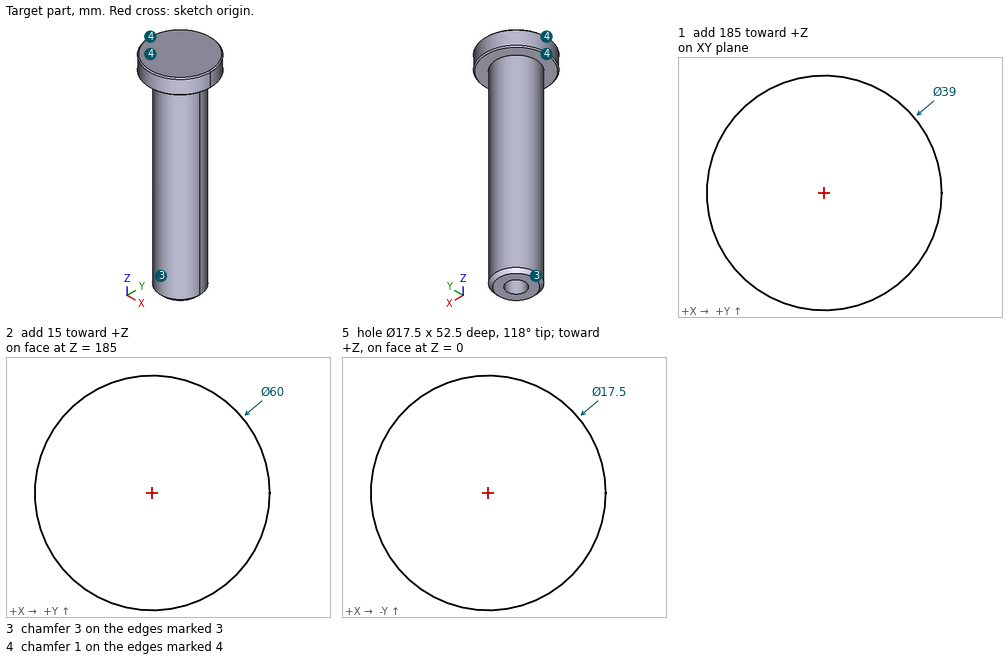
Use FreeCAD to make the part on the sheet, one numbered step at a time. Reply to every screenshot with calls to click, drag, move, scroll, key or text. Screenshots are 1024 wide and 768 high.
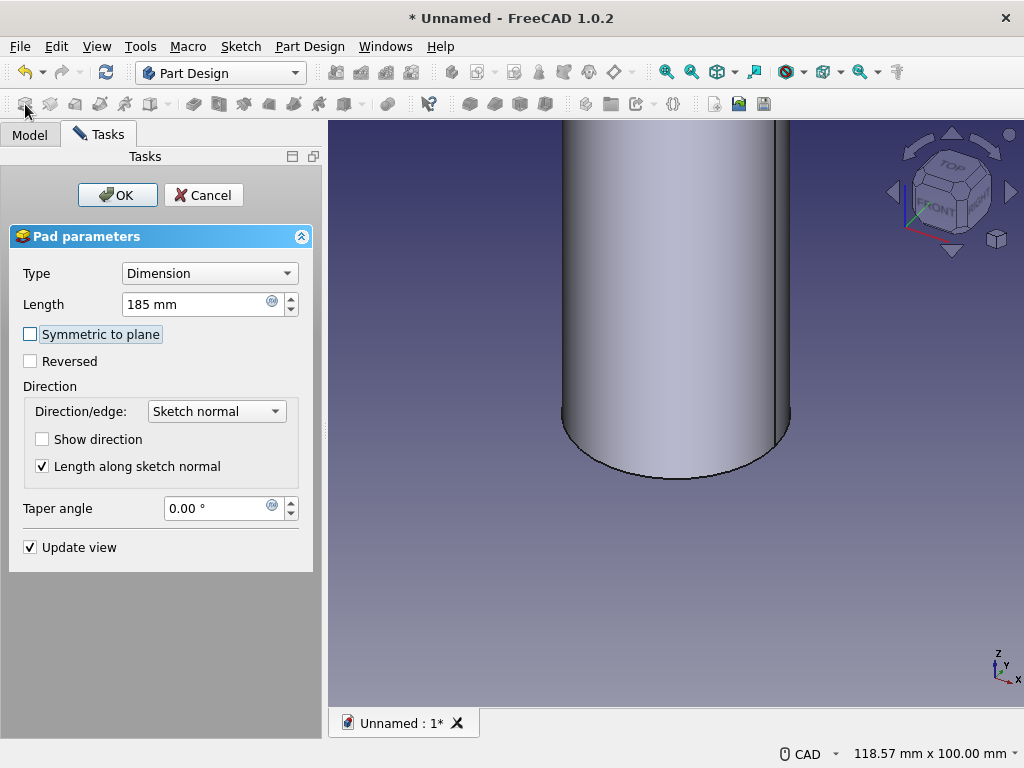
click(118, 195)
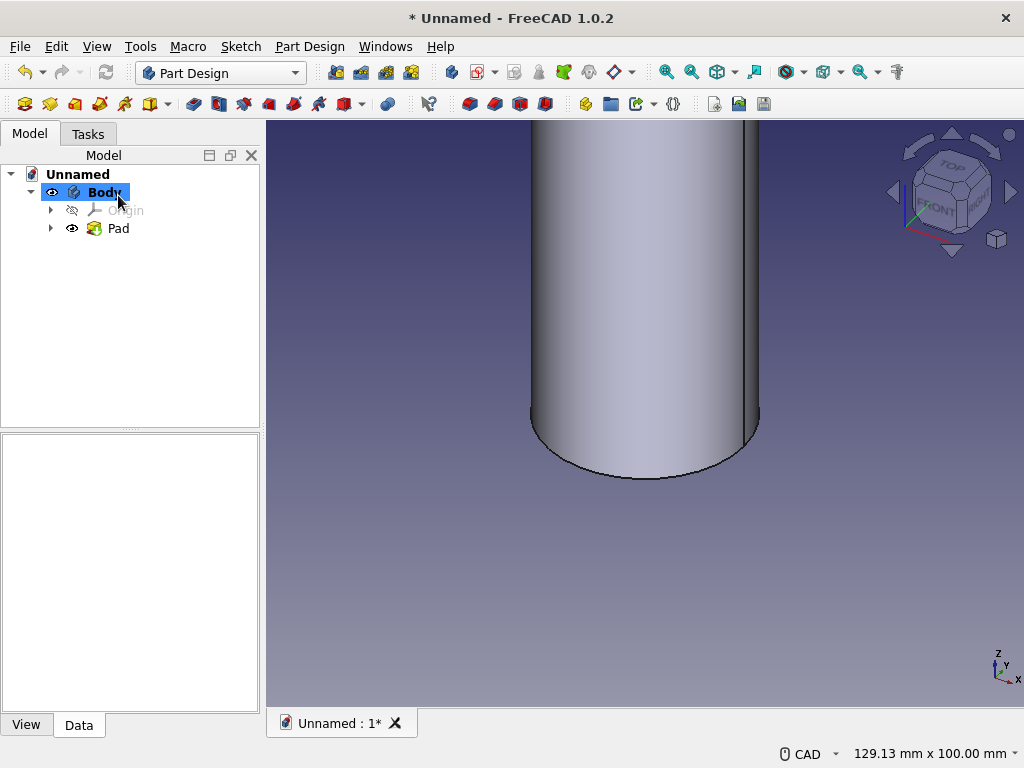
click(667, 72)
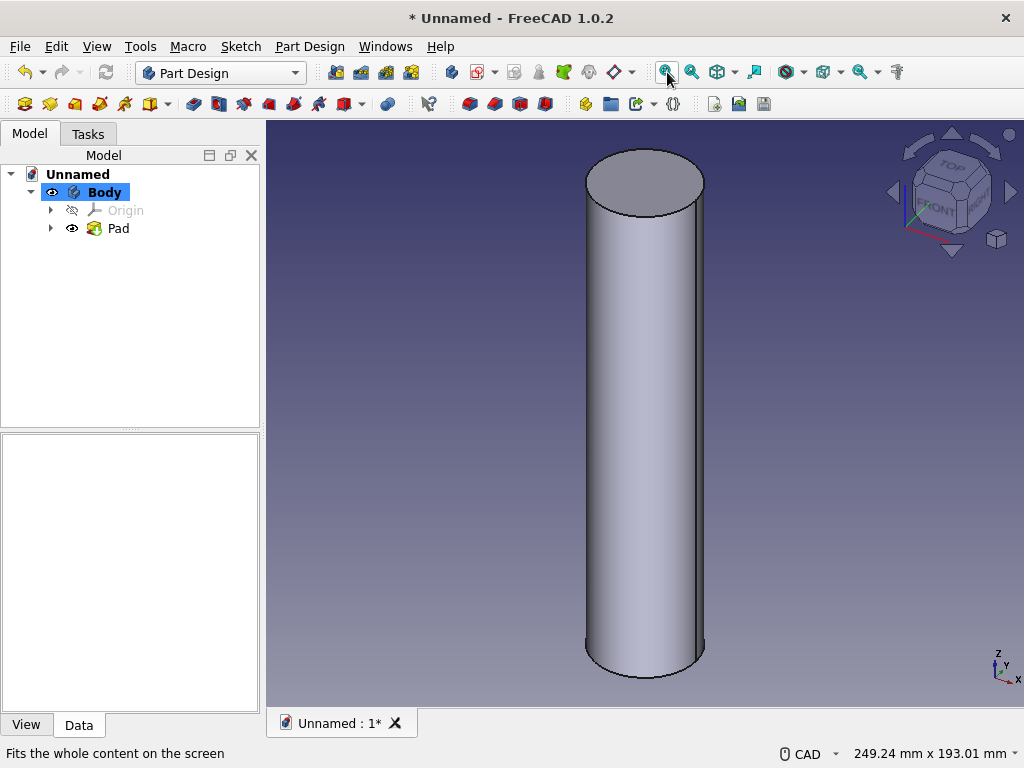
click(645, 182)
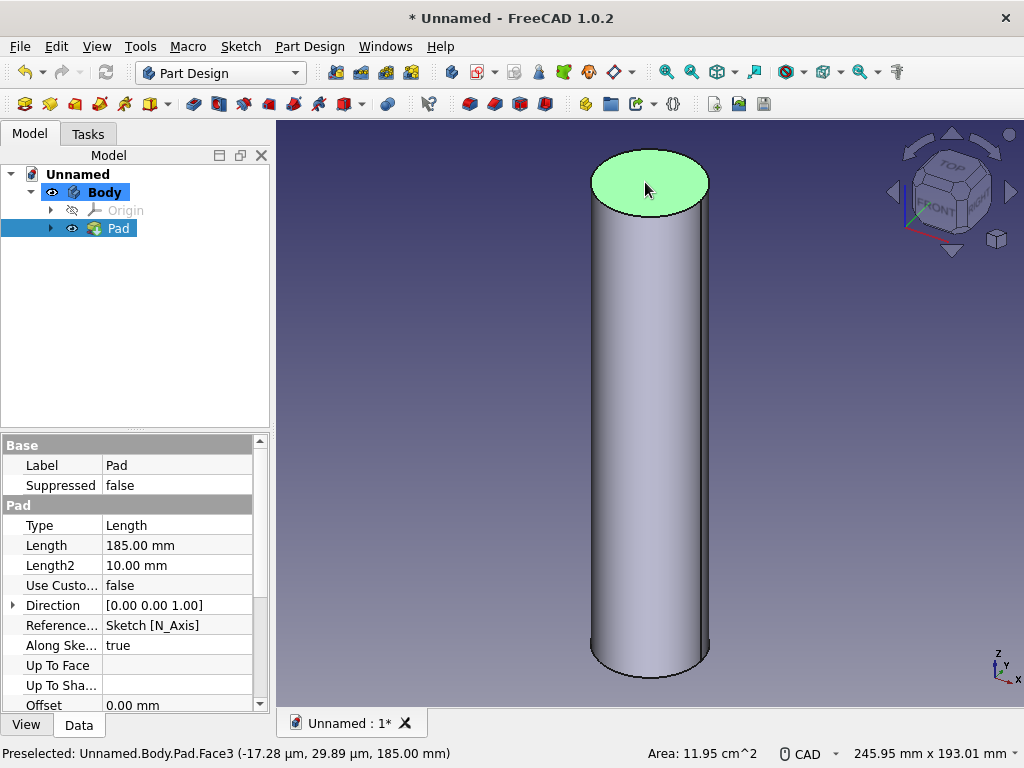
click(476, 72)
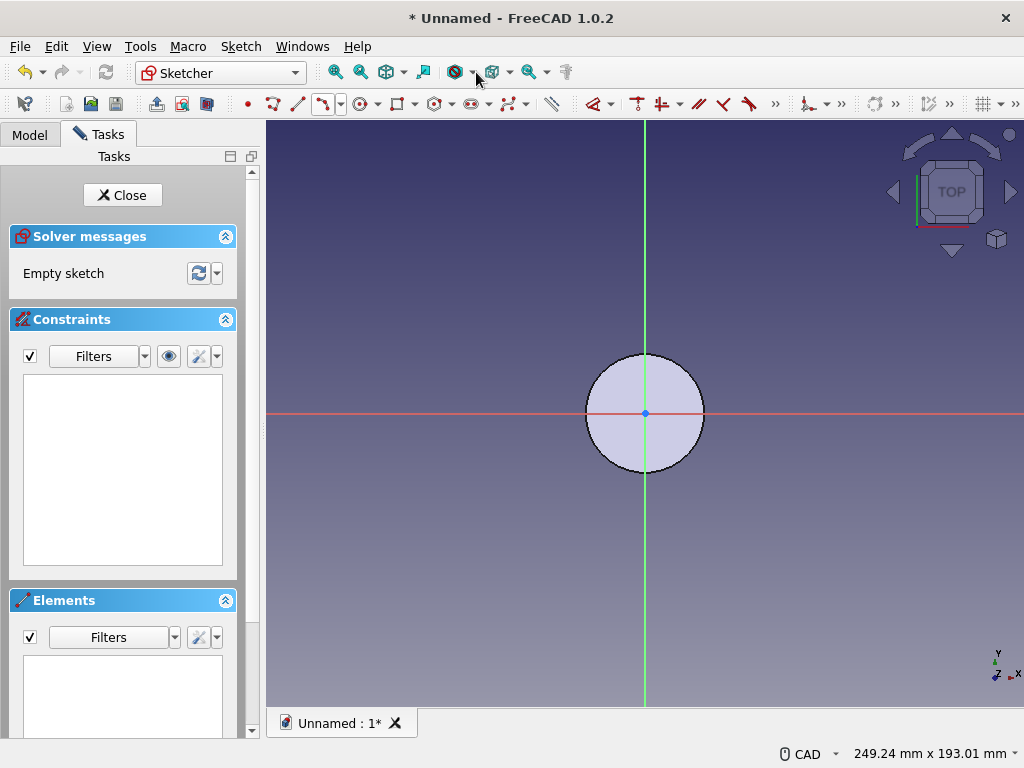
scroll(701, 413, up, 4)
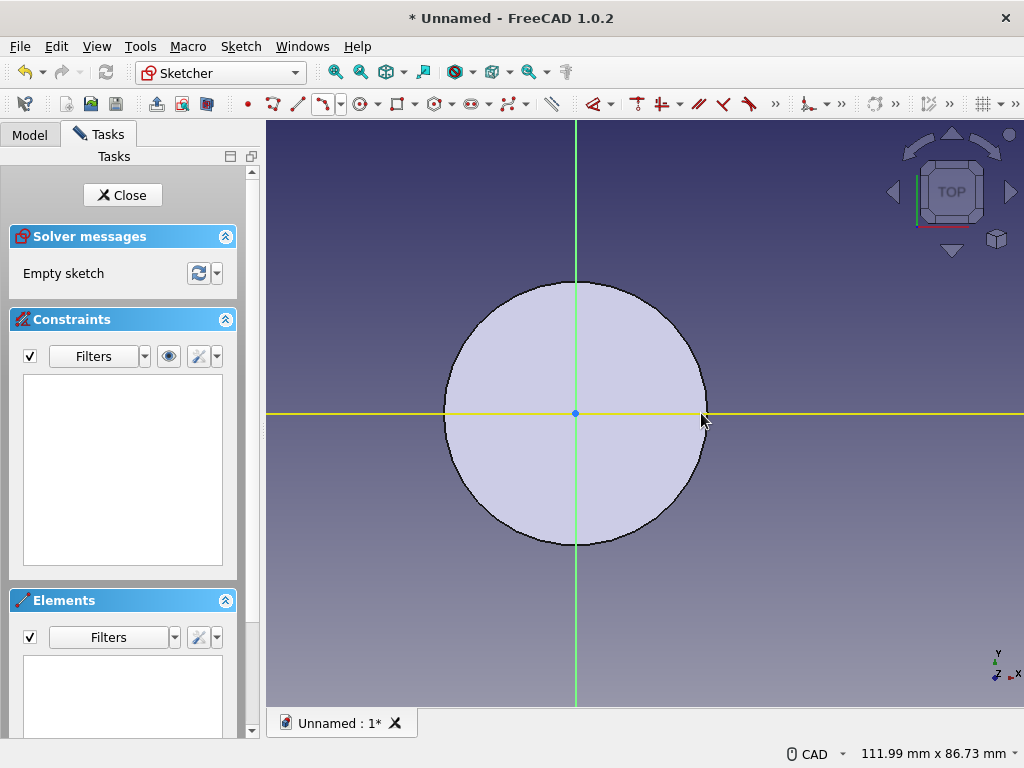
click(360, 104)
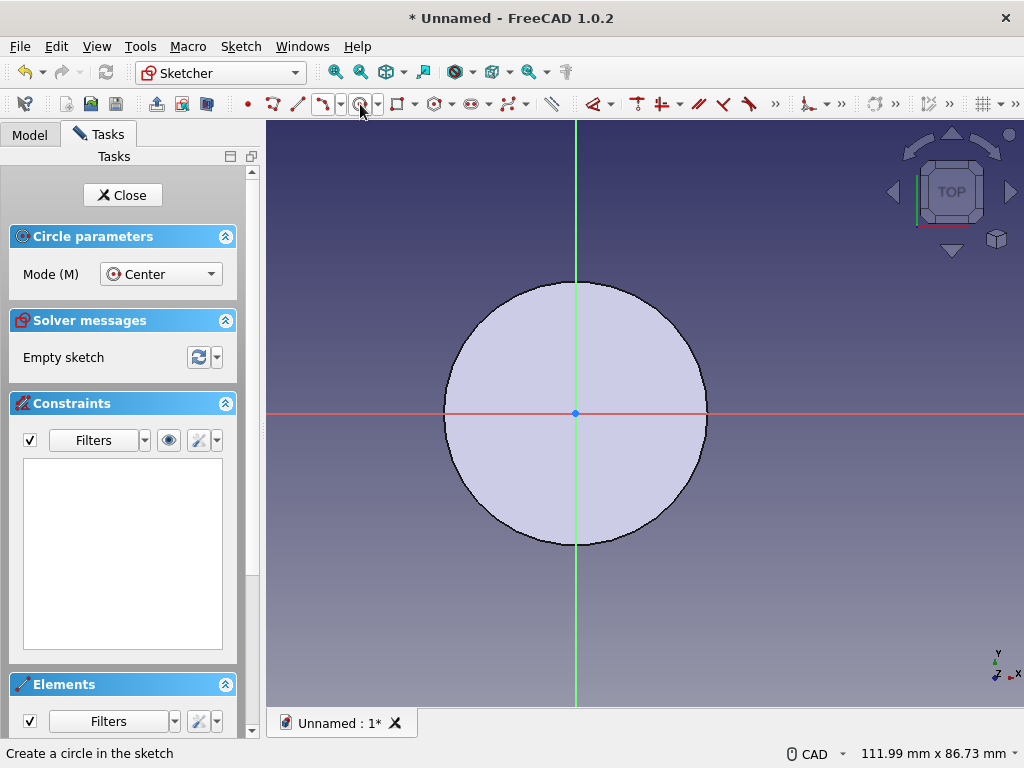
click(576, 414)
click(719, 270)
key(Escape)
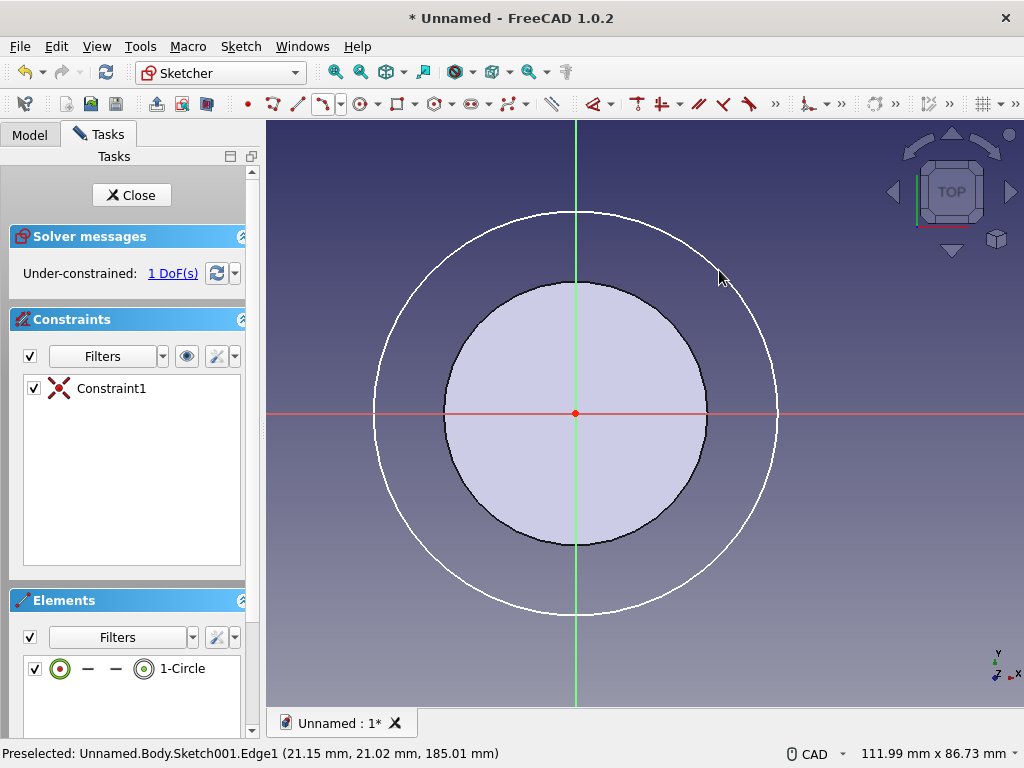
click(592, 104)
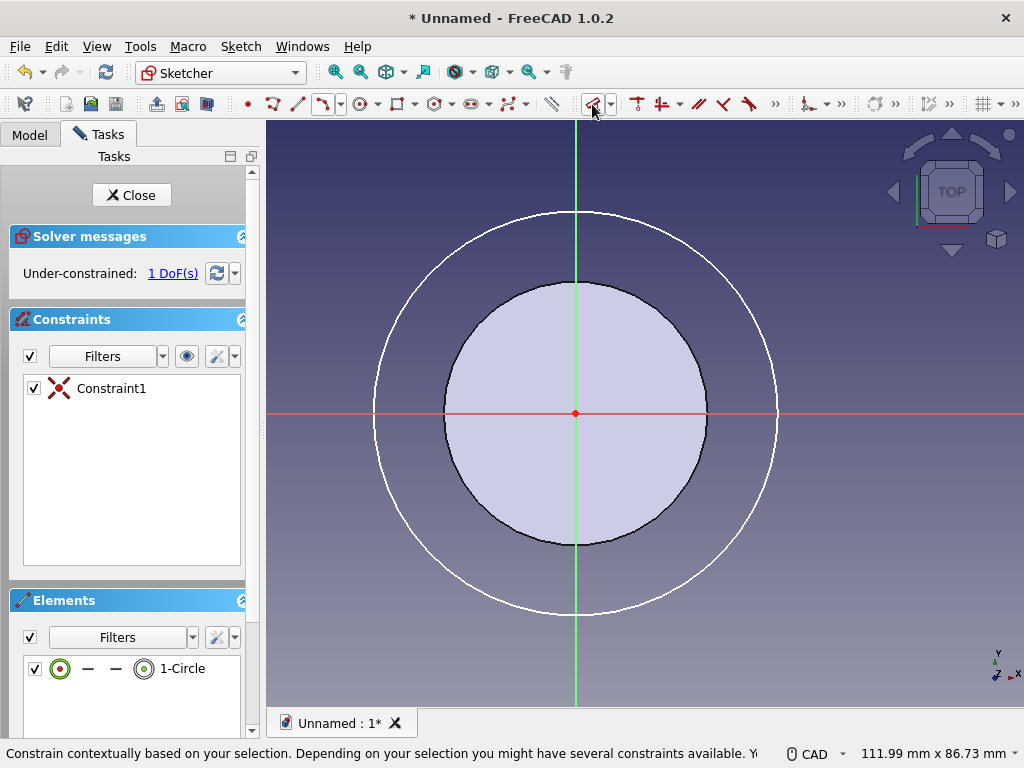
click(718, 270)
click(741, 247)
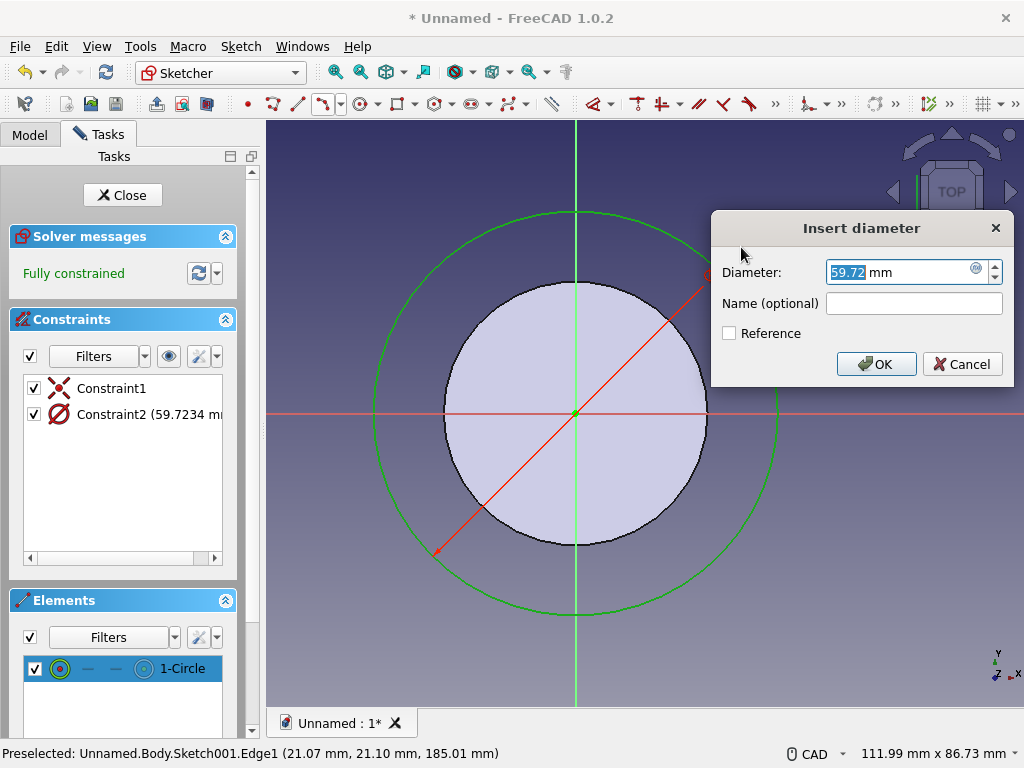
text(60)
key(Return)
key(Escape)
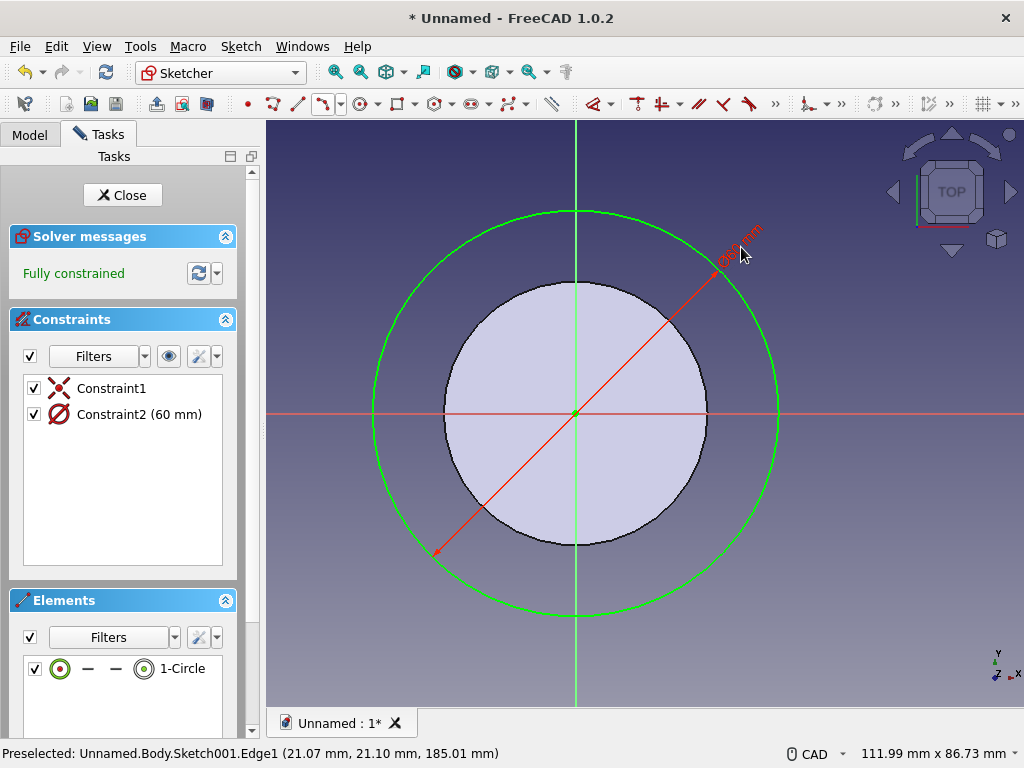
click(123, 195)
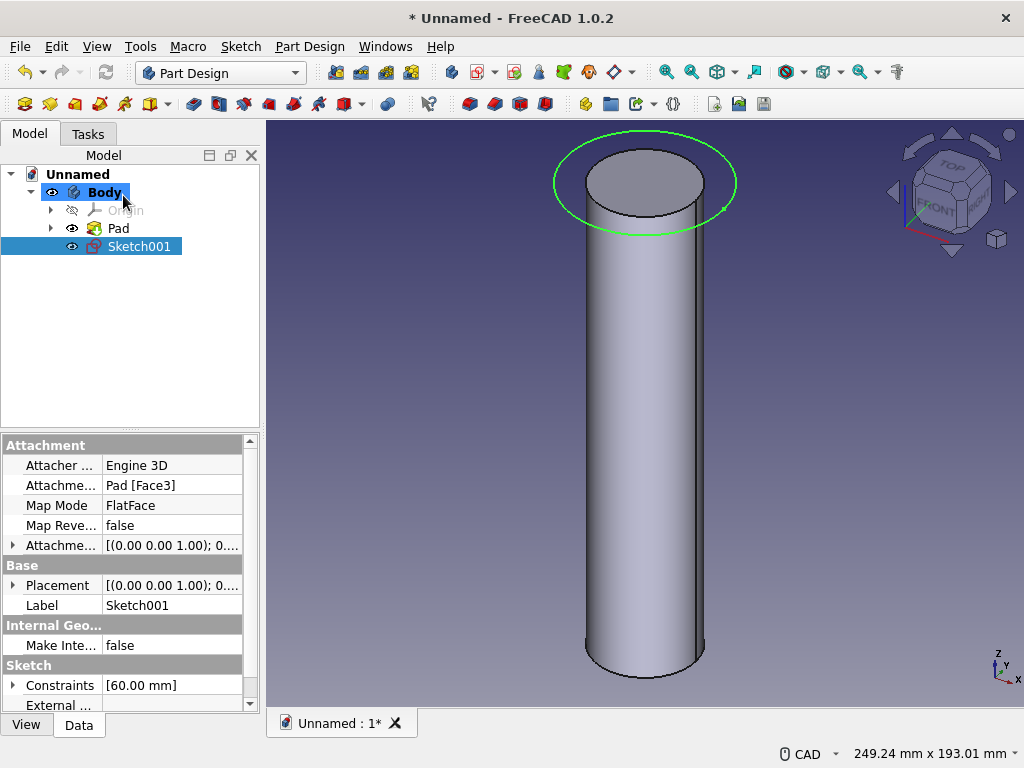
click(25, 104)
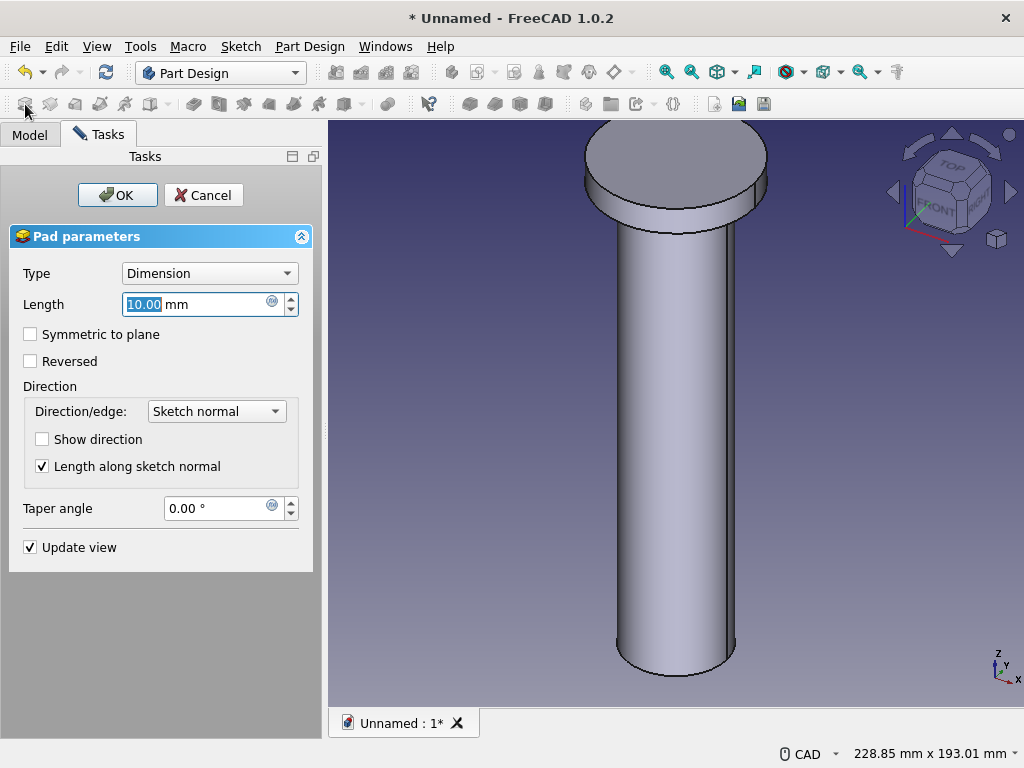
text(15)
key(Tab)